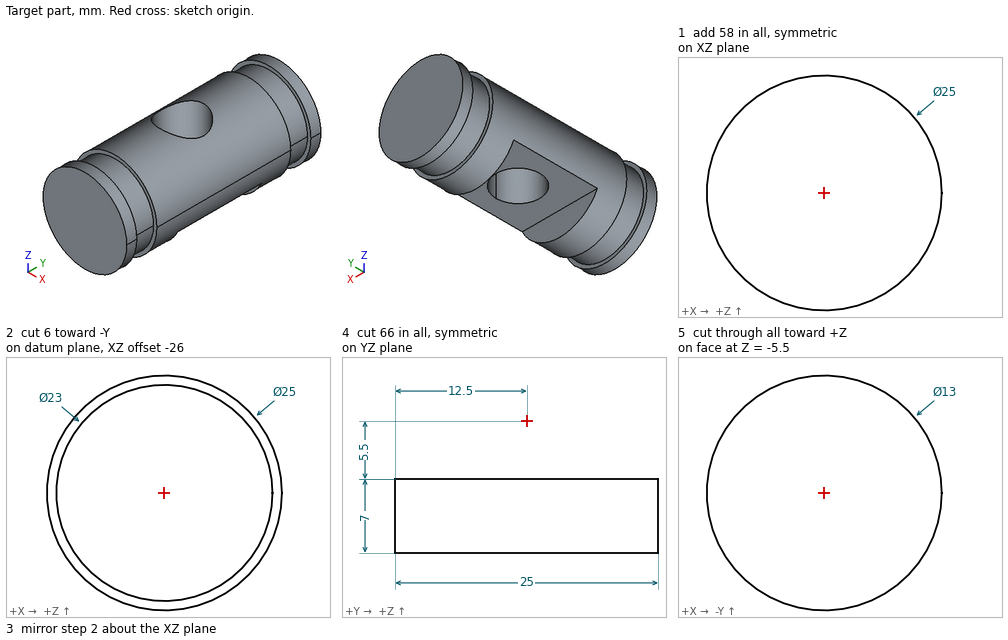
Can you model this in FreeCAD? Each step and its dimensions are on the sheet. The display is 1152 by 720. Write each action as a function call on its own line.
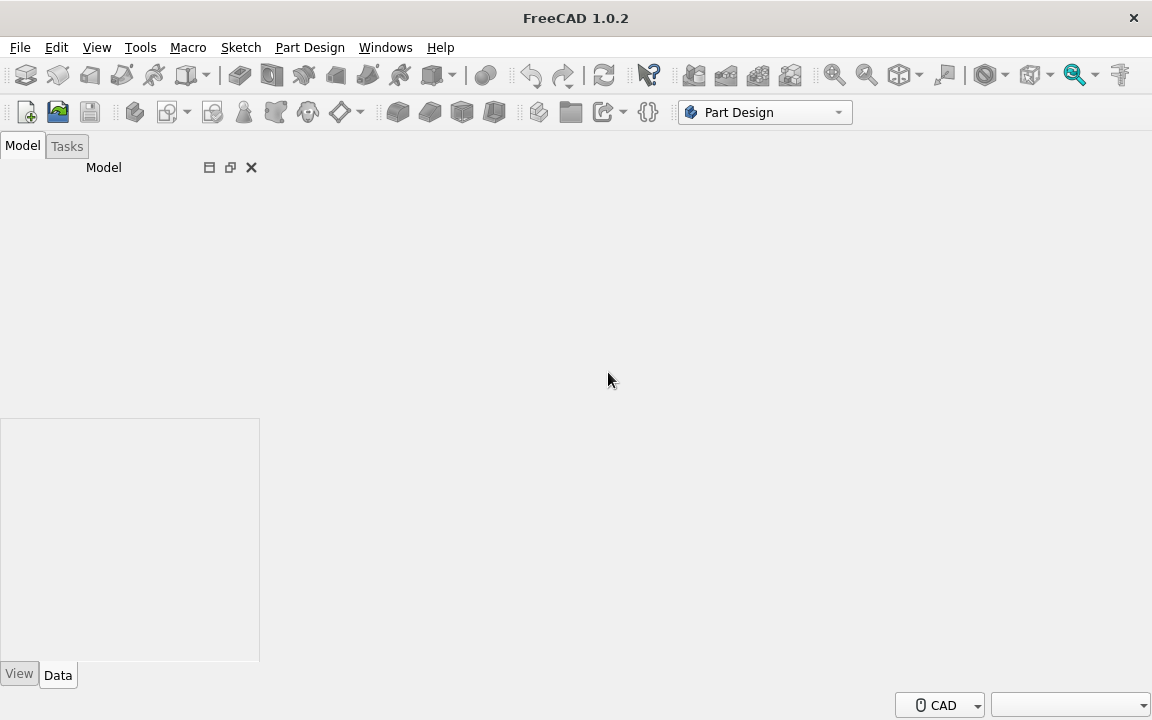
click(26, 112)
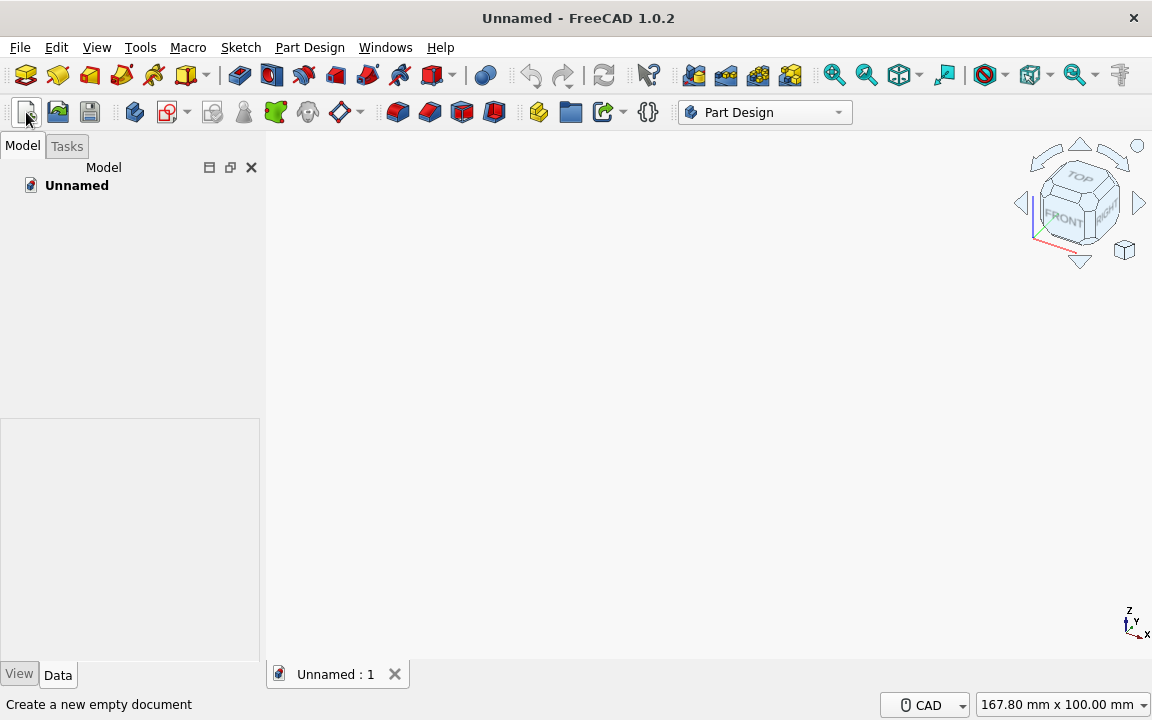
click(168, 112)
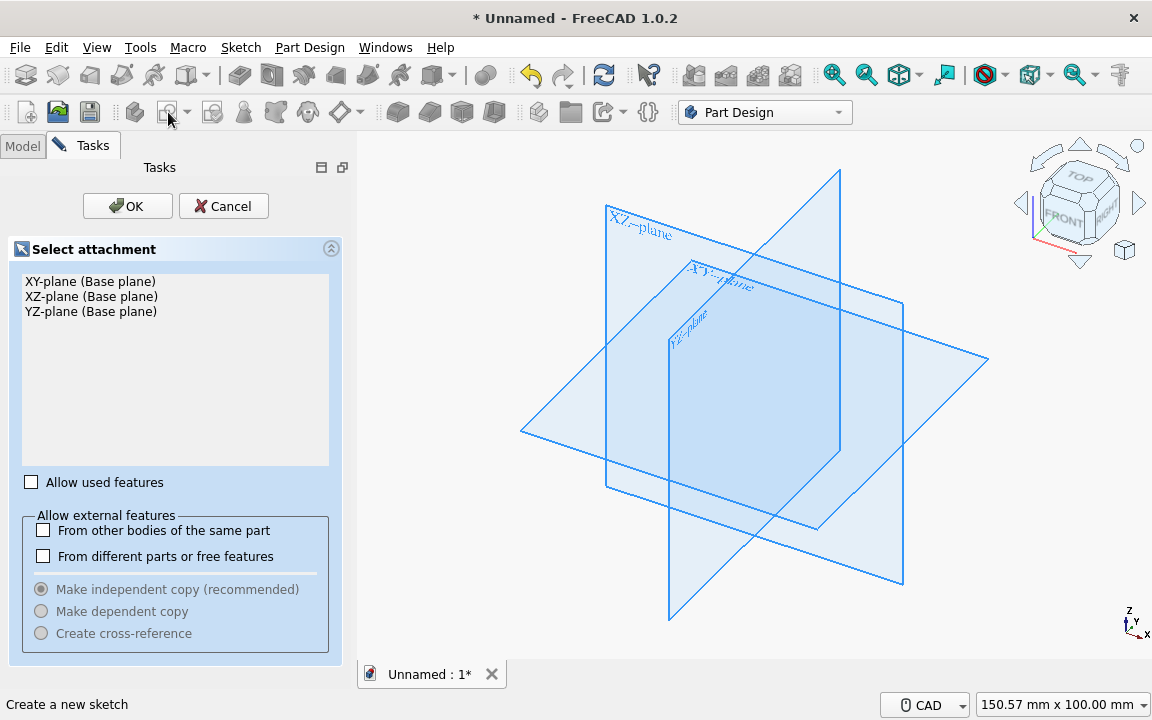
click(82, 296)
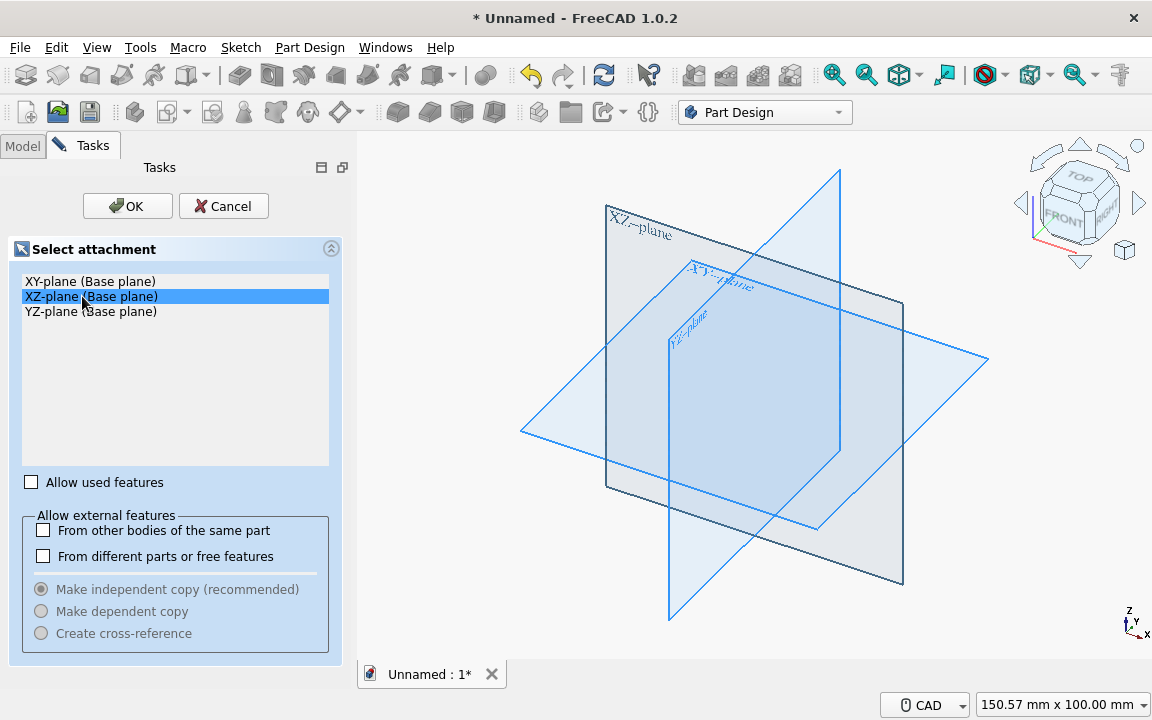
click(128, 206)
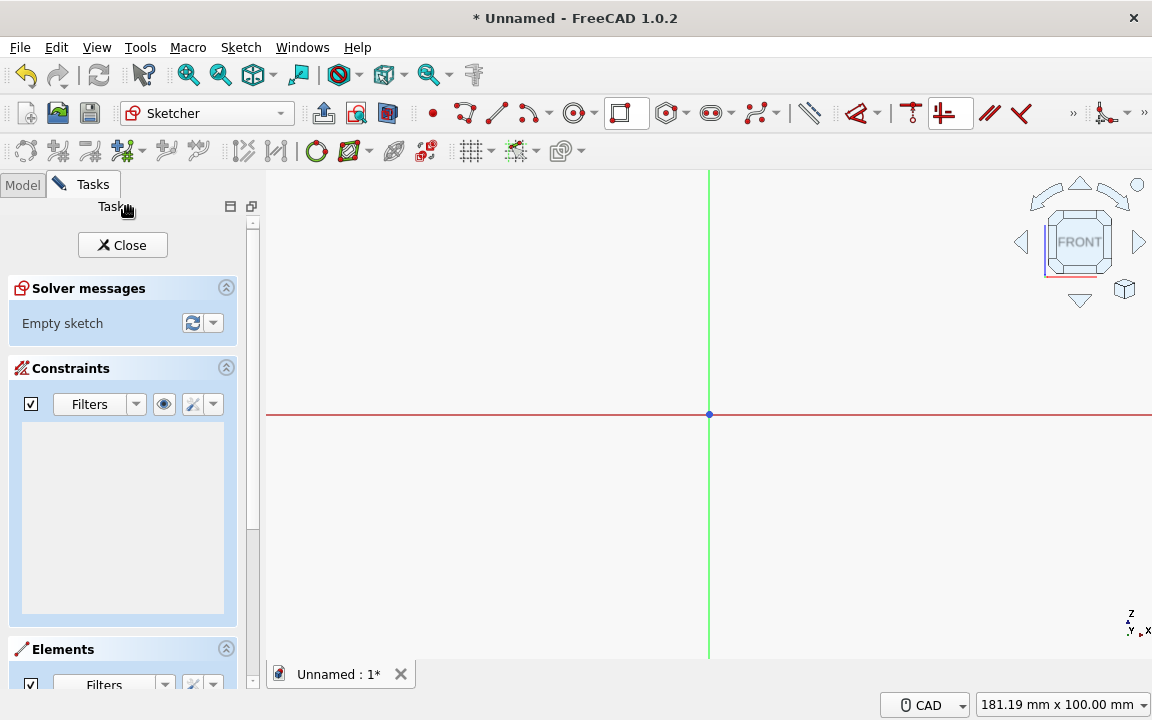
scroll(749, 415, up, 5)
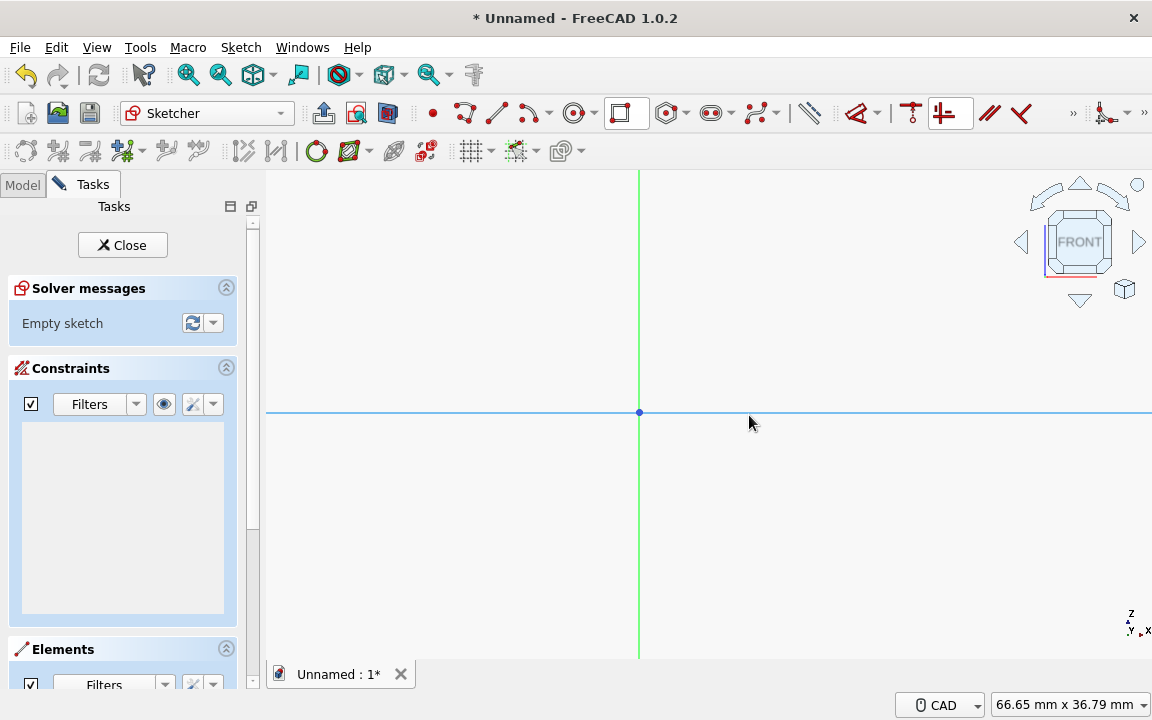
click(574, 114)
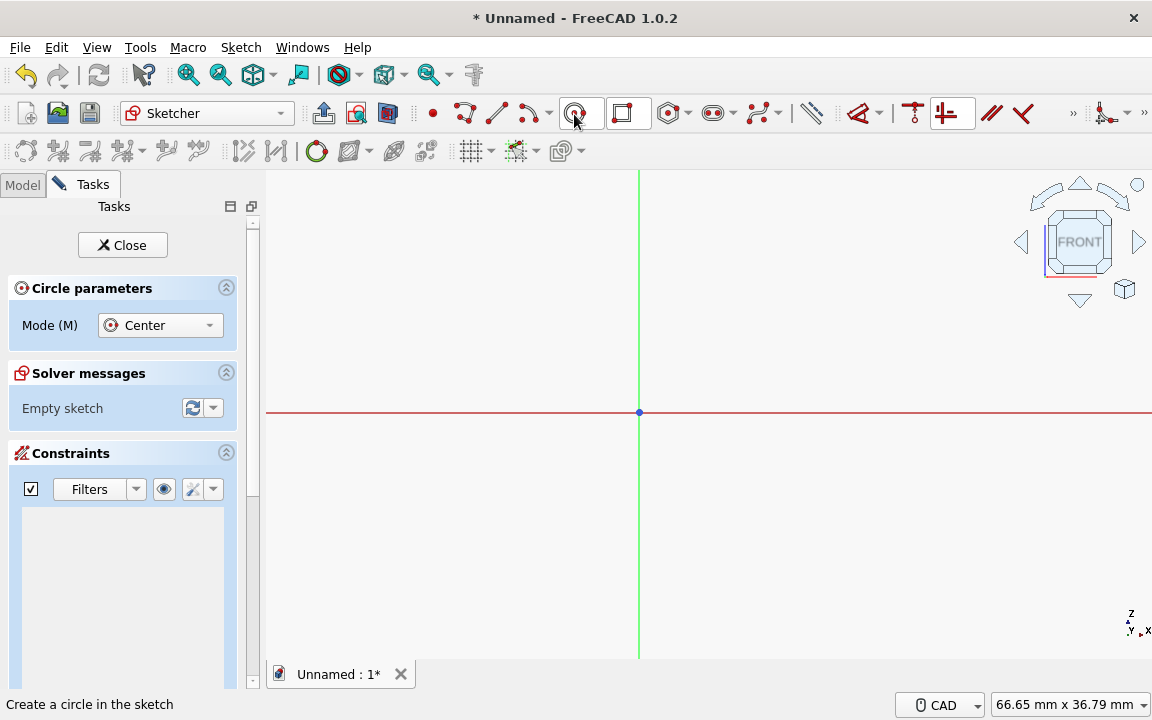
click(639, 413)
click(757, 295)
key(Escape)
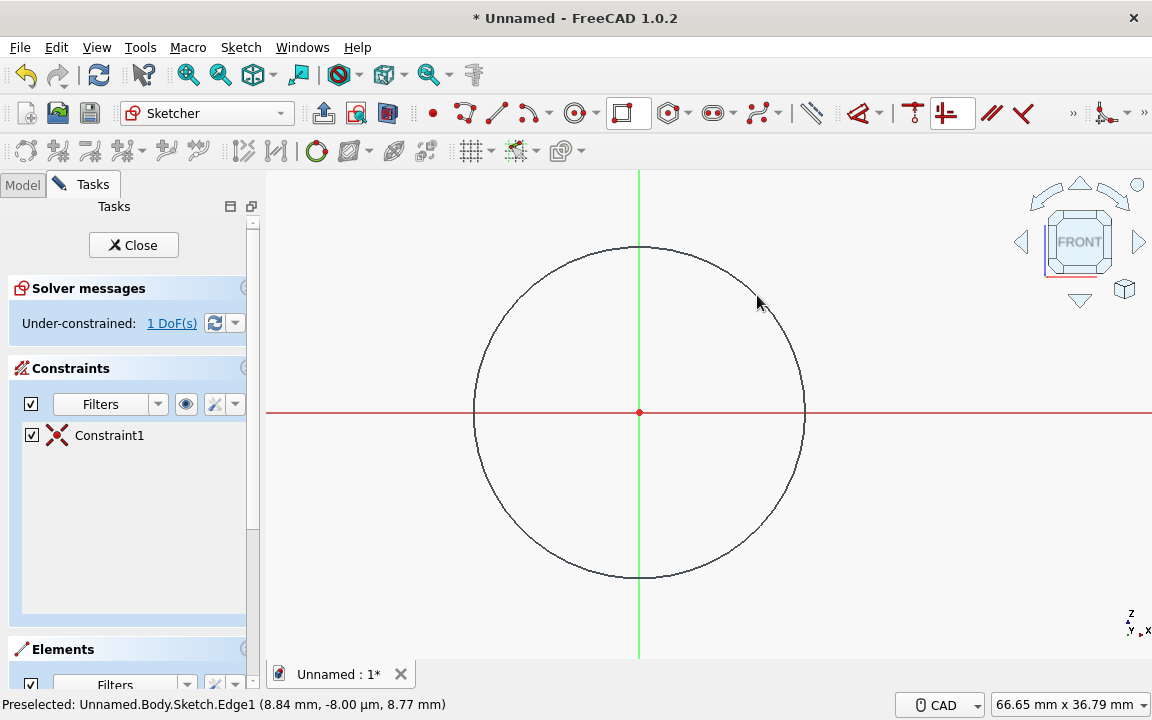
click(858, 114)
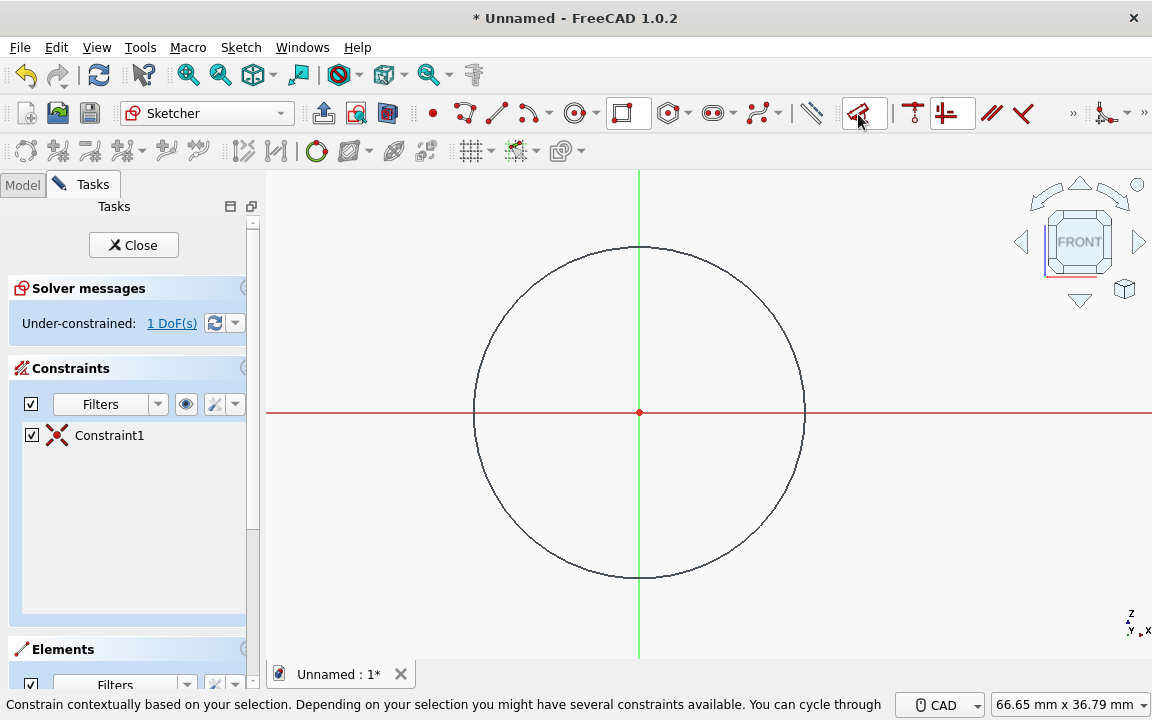
click(756, 295)
click(779, 272)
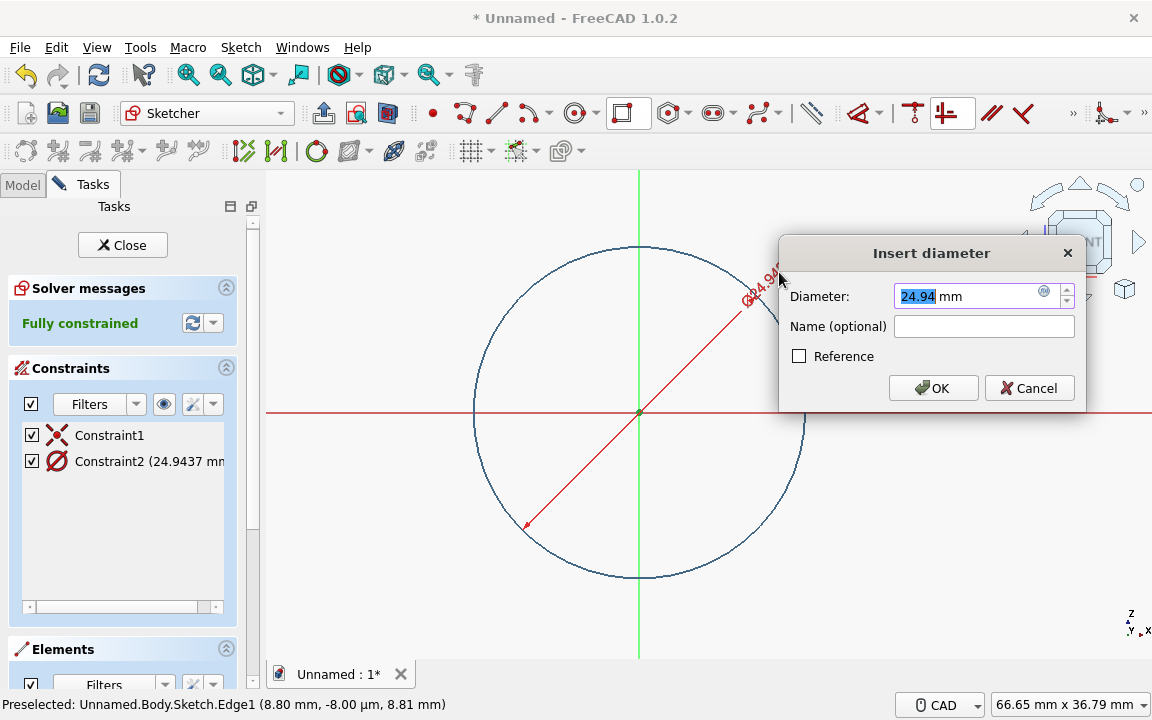
text(25)
key(Return)
key(Escape)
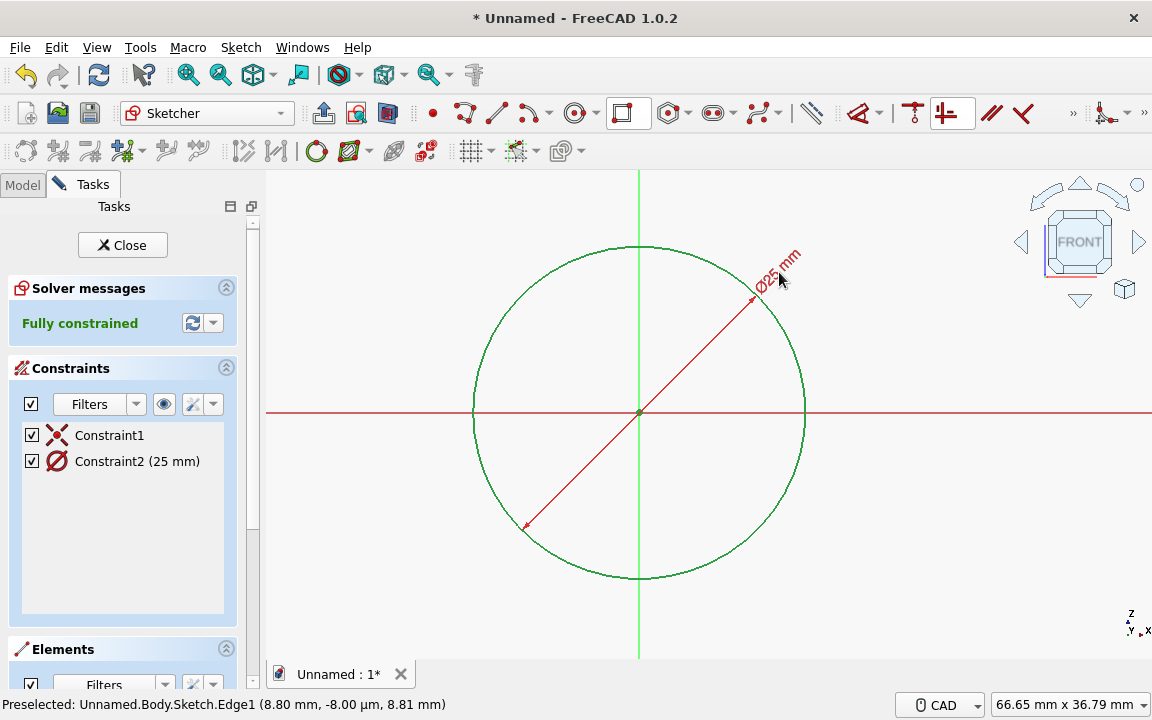
click(123, 245)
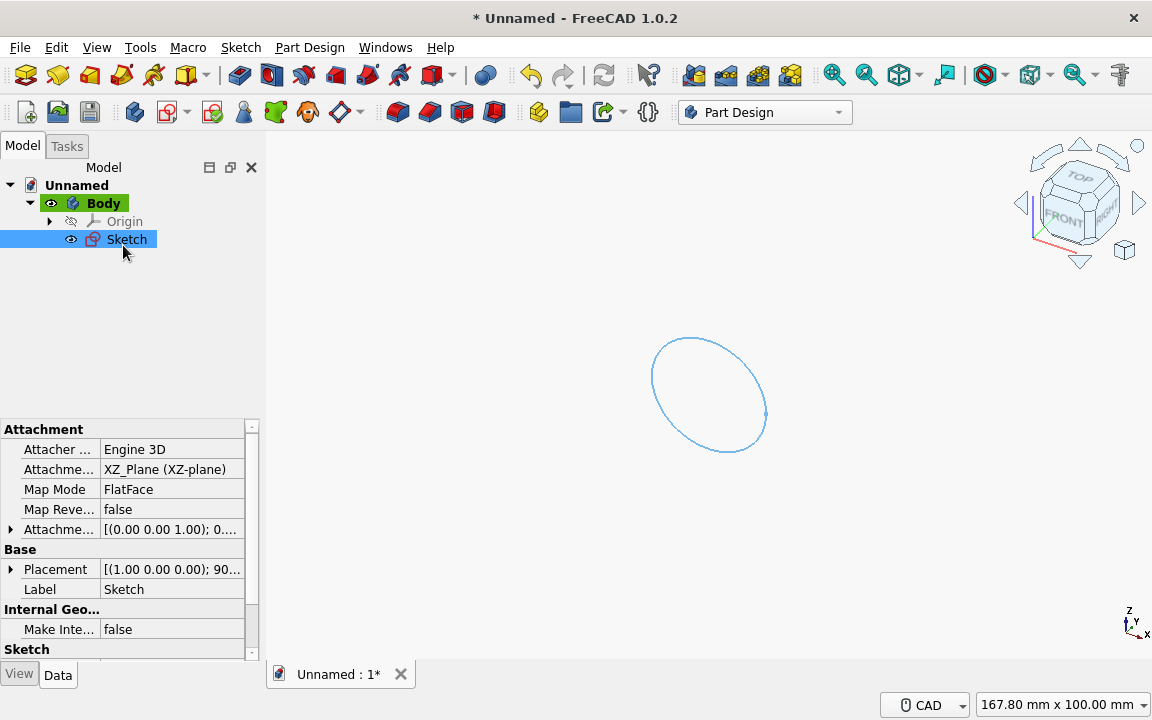
click(26, 76)